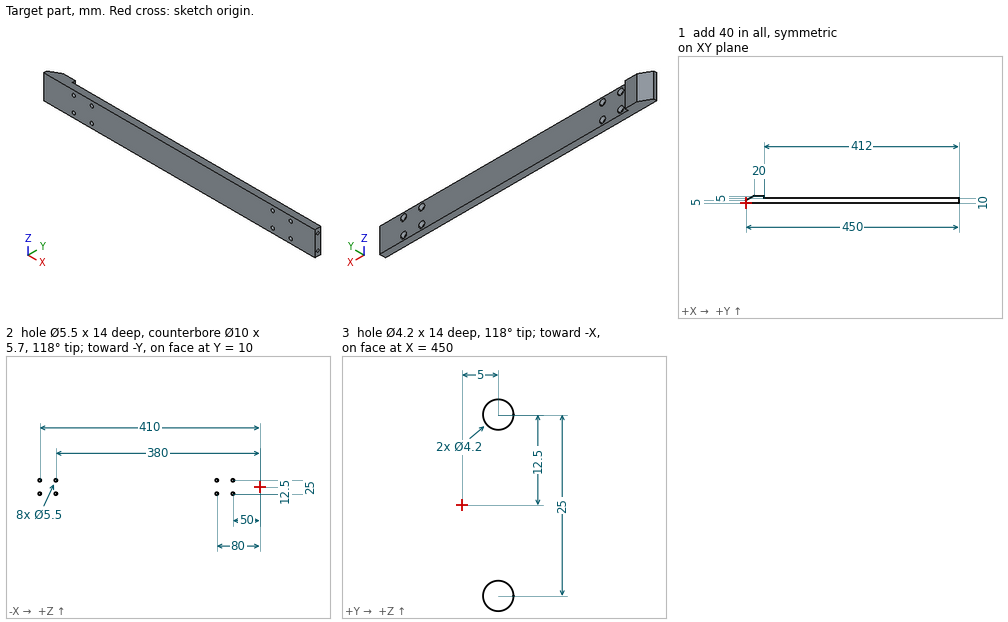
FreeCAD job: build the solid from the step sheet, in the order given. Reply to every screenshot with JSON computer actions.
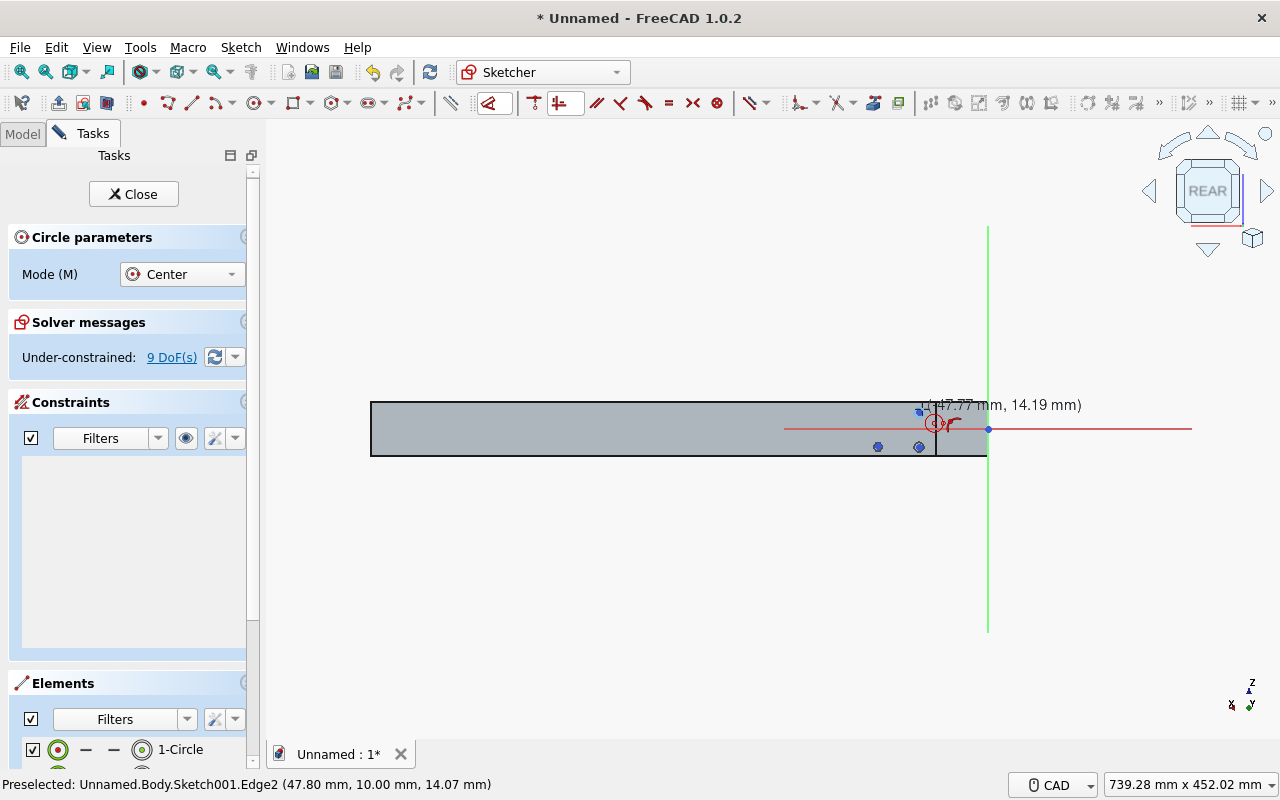
{"action": "left_click", "coordinate": [878, 412]}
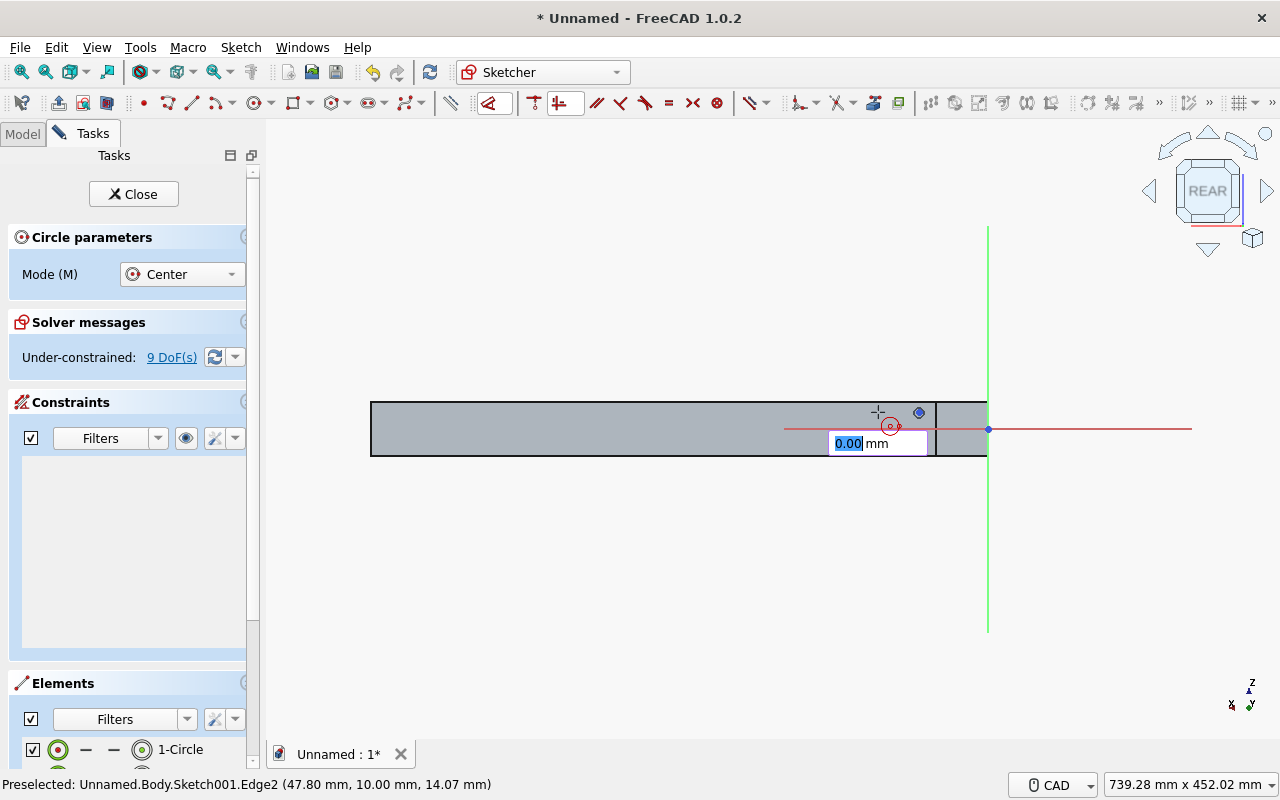
{"action": "scroll", "coordinate": [881, 409], "scroll_direction": "up", "scroll_amount": 8}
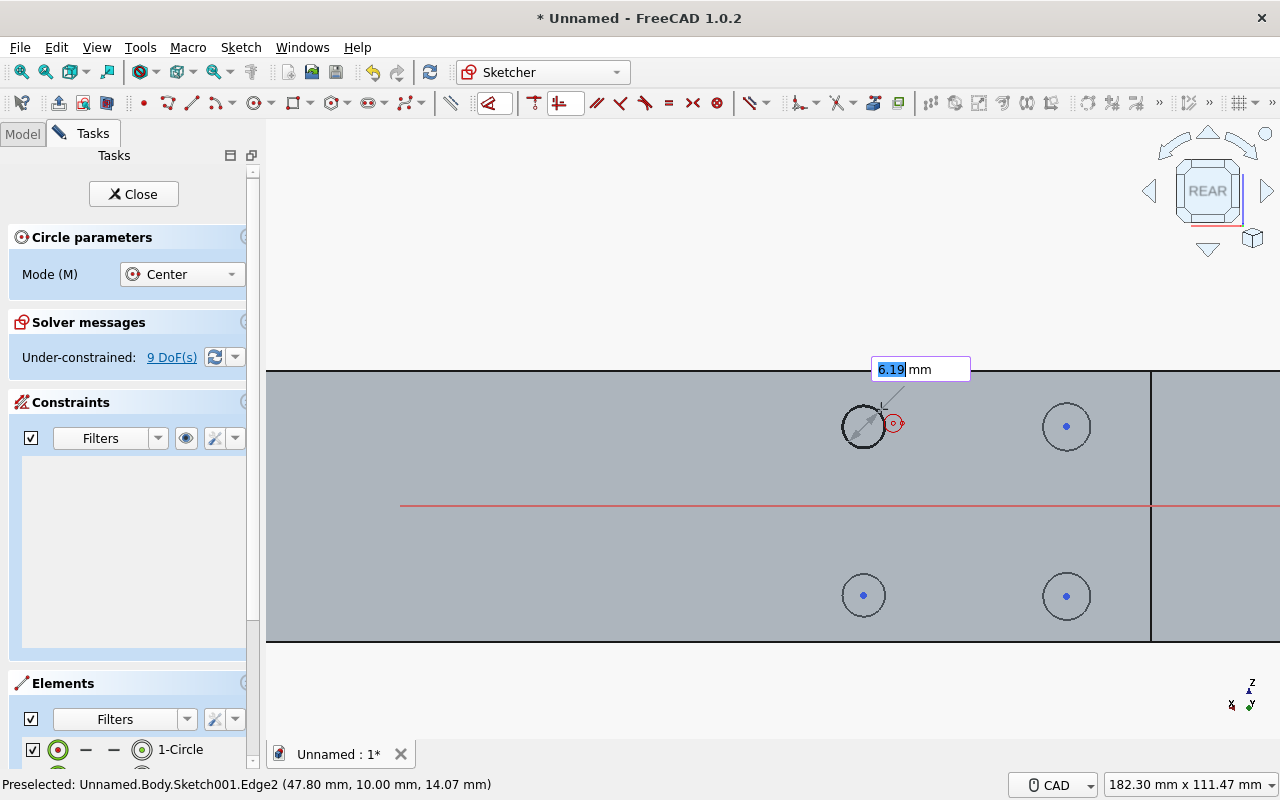
{"action": "left_click", "coordinate": [878, 408]}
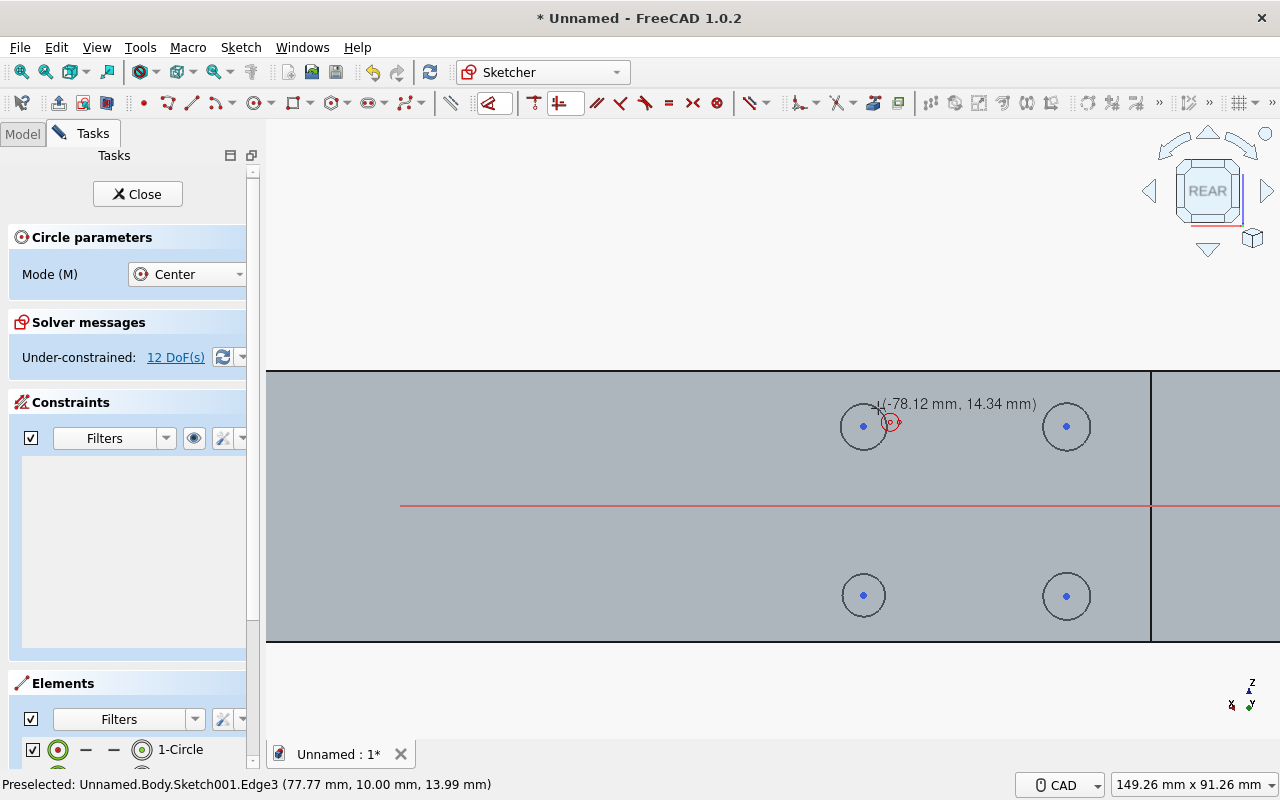
{"action": "scroll", "coordinate": [881, 409], "scroll_direction": "down", "scroll_amount": 8}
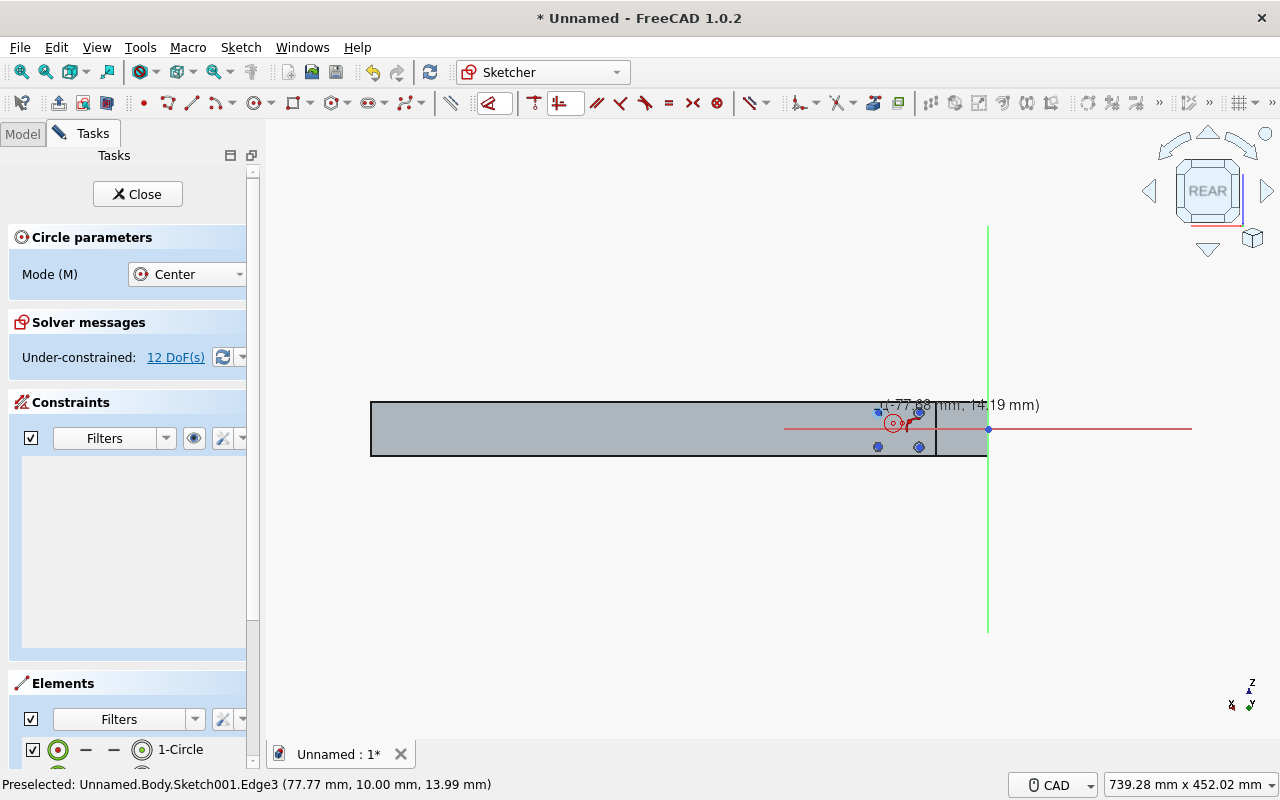
{"action": "scroll", "coordinate": [467, 412], "scroll_direction": "up", "scroll_amount": 9}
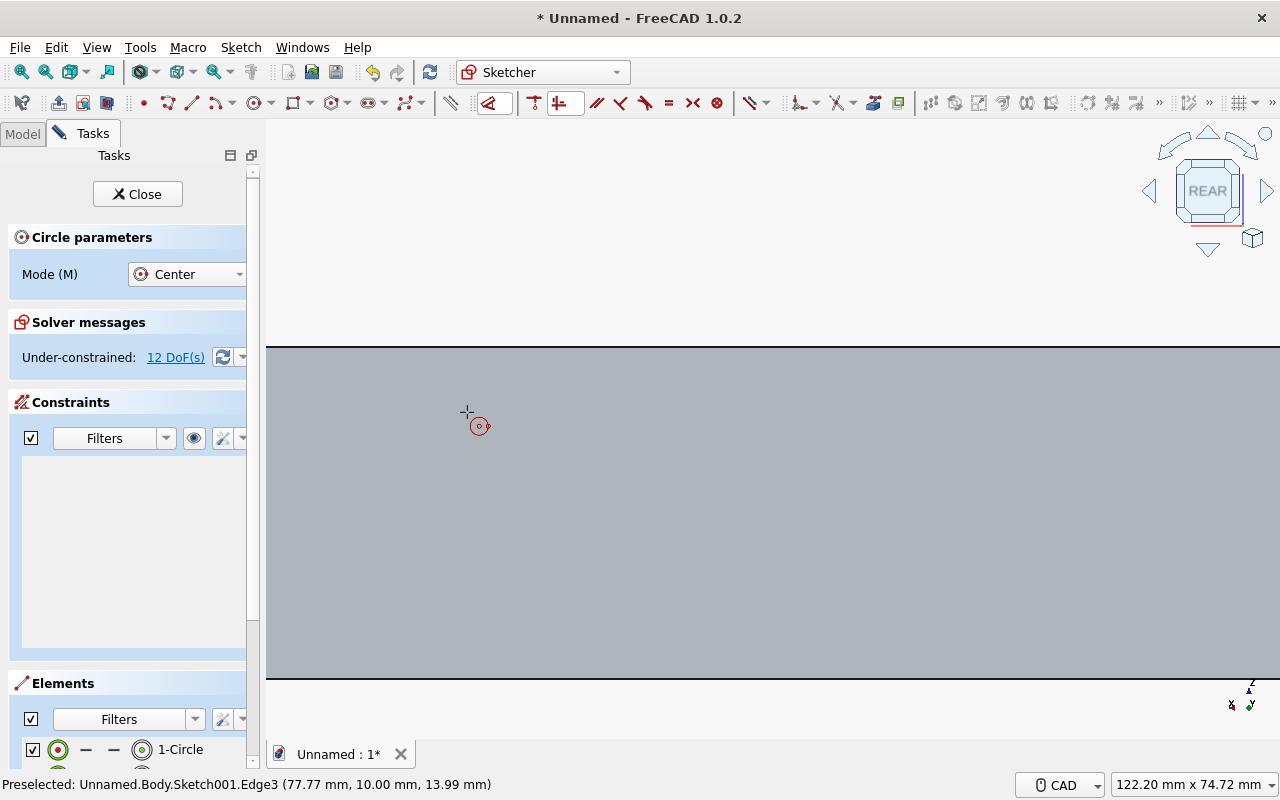
{"action": "scroll", "coordinate": [467, 412], "scroll_direction": "down", "scroll_amount": 9}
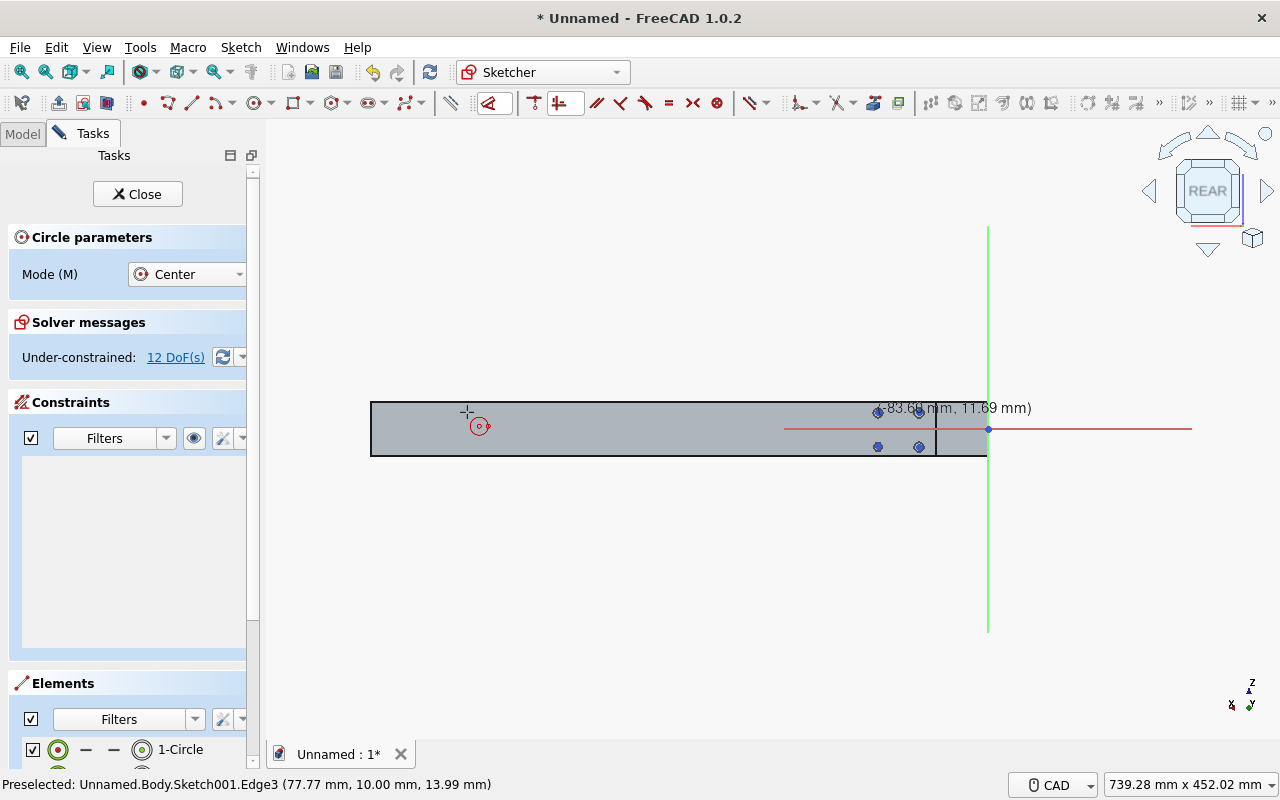
{"action": "left_click", "coordinate": [467, 412]}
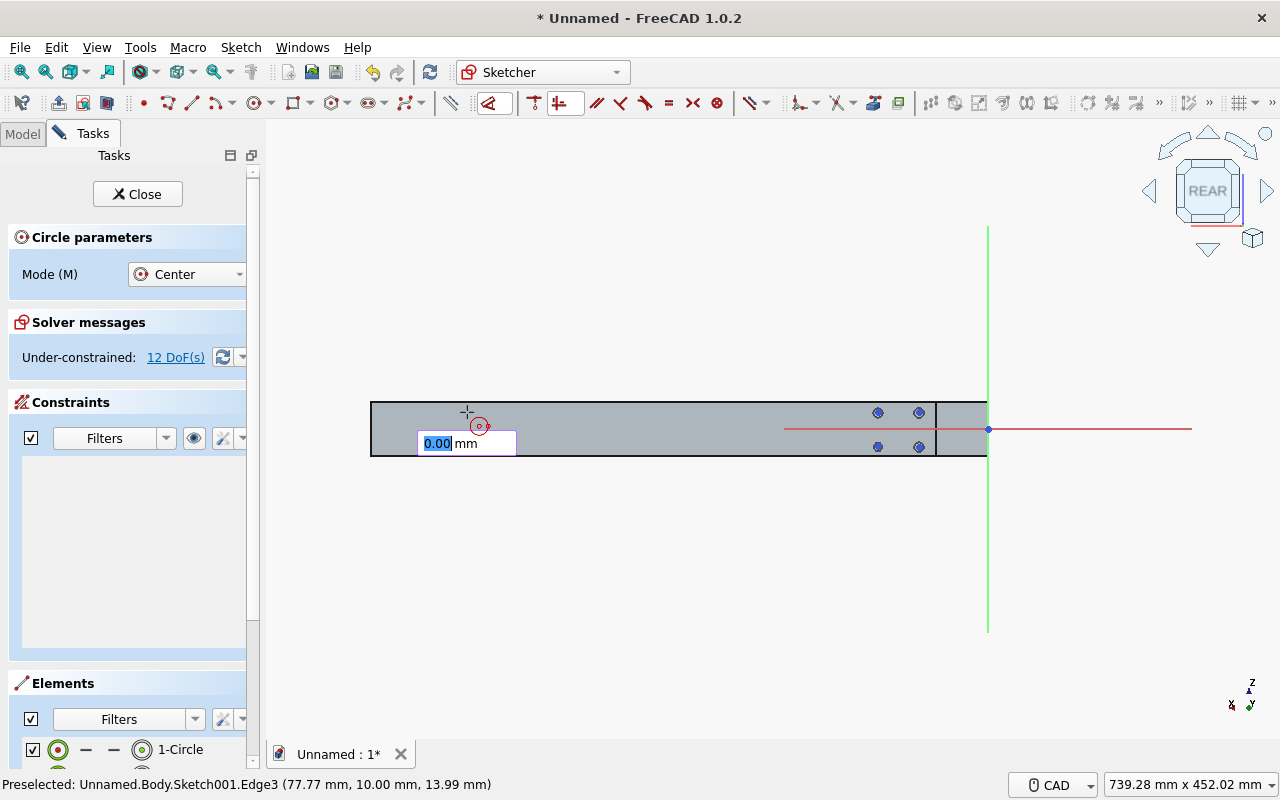
{"action": "scroll", "coordinate": [469, 409], "scroll_direction": "up", "scroll_amount": 8}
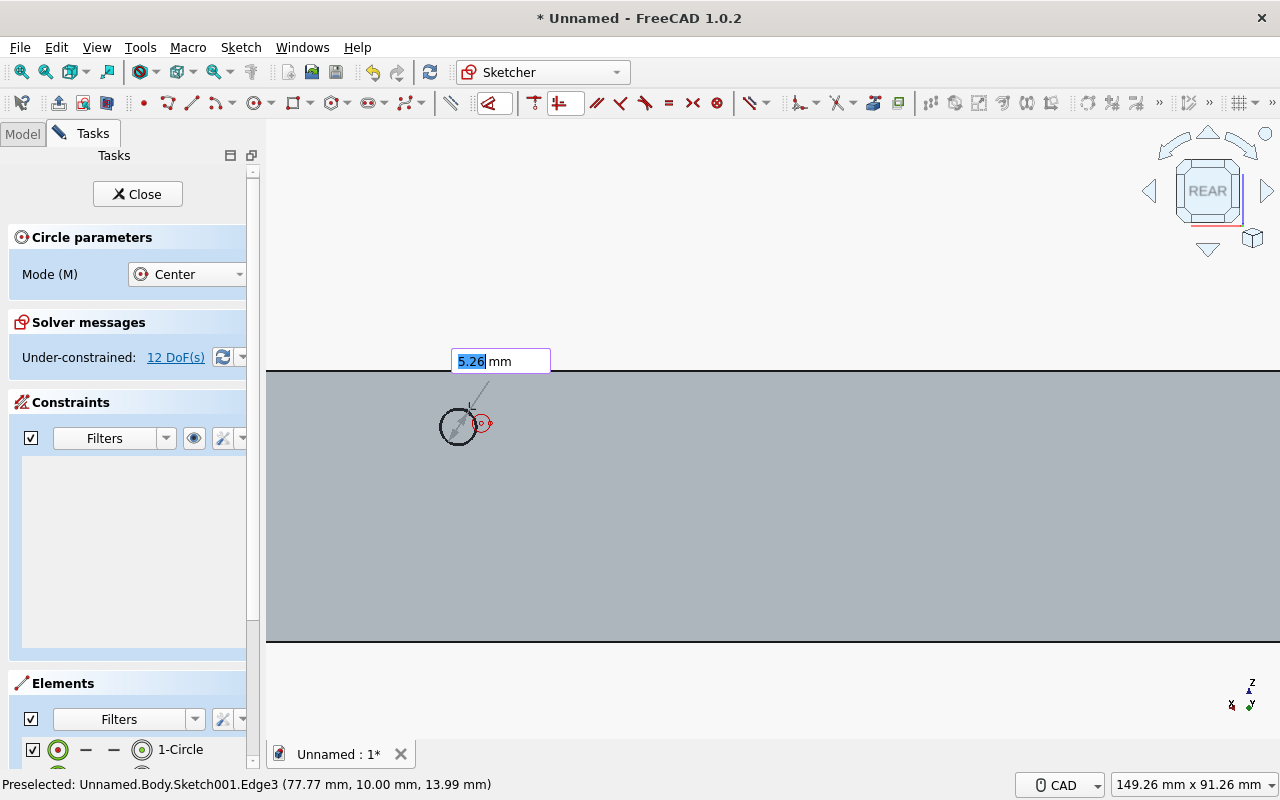
{"action": "left_click", "coordinate": [471, 408]}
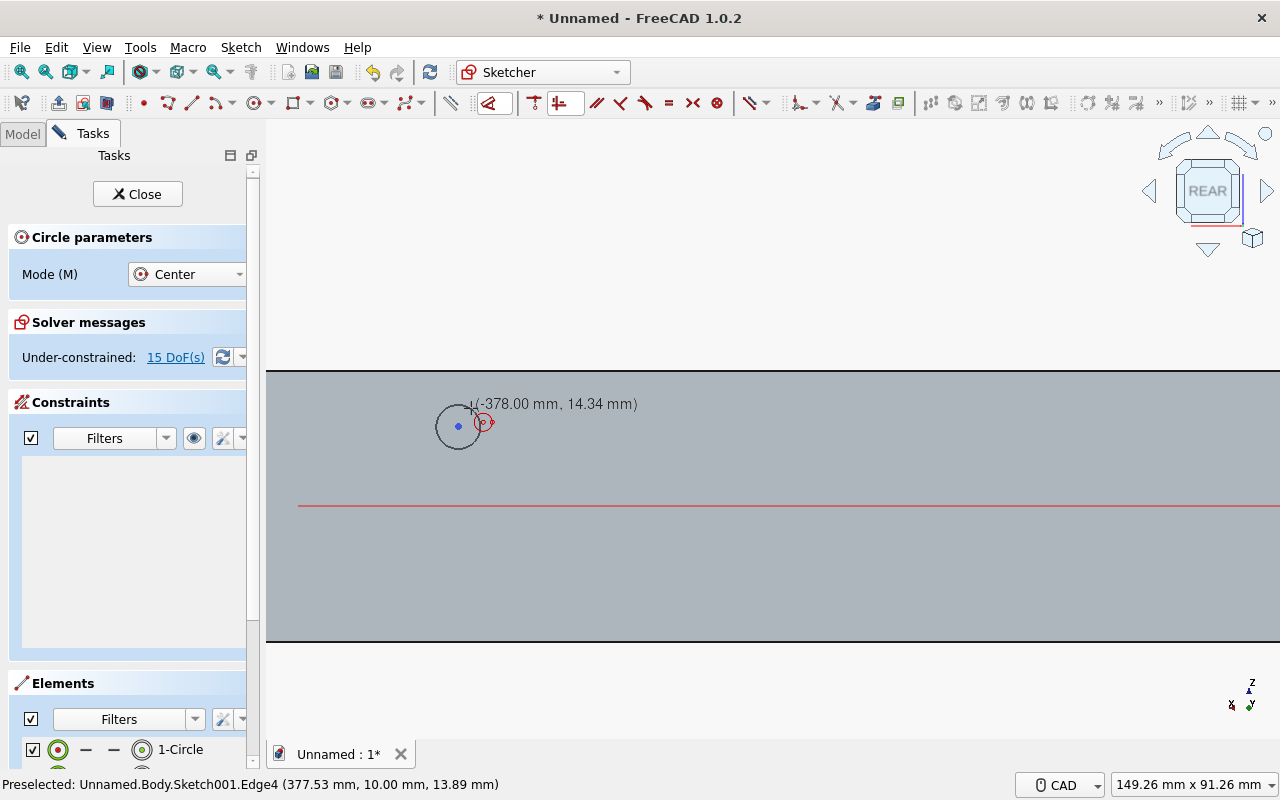
{"action": "scroll", "coordinate": [469, 409], "scroll_direction": "down", "scroll_amount": 8}